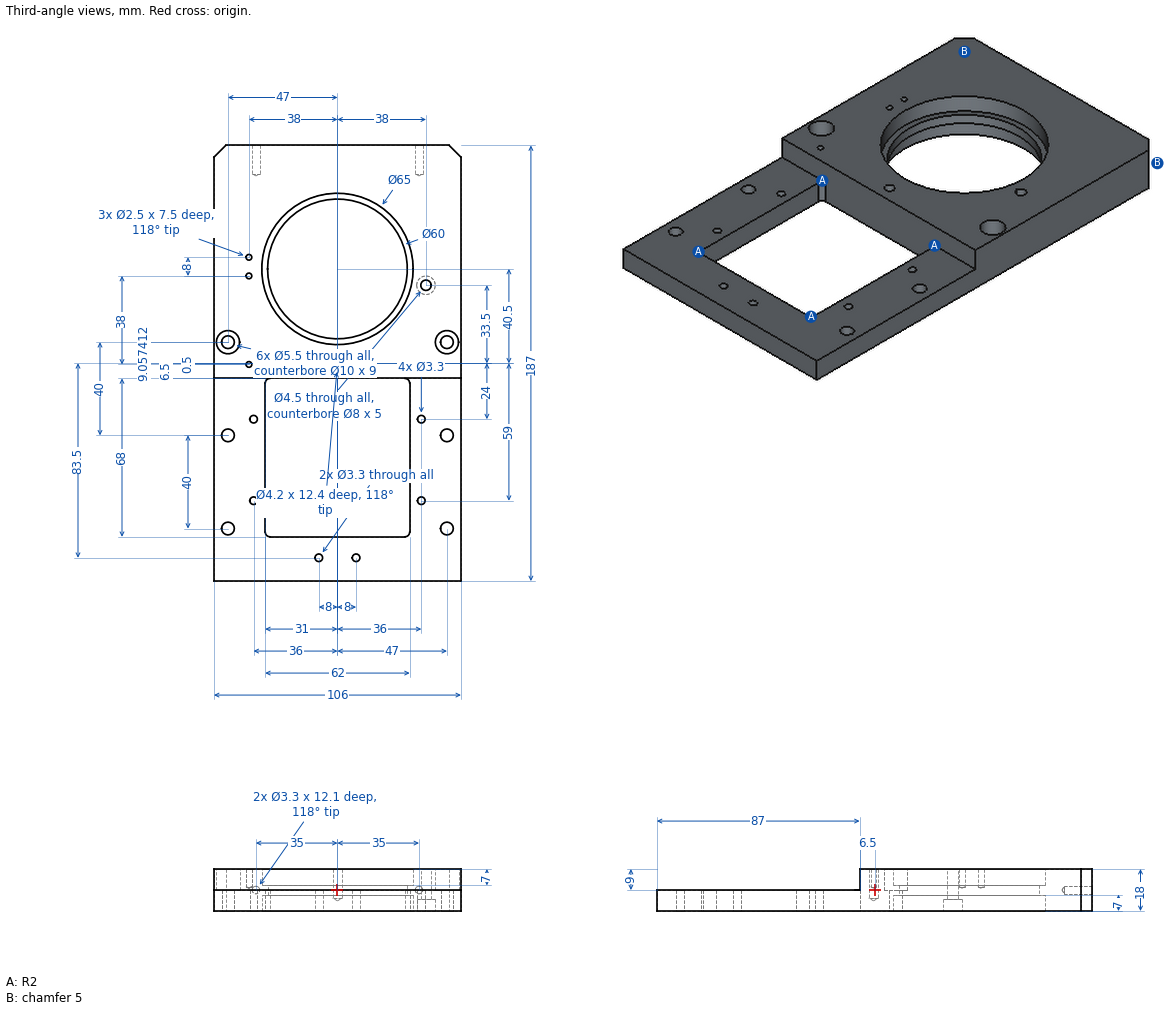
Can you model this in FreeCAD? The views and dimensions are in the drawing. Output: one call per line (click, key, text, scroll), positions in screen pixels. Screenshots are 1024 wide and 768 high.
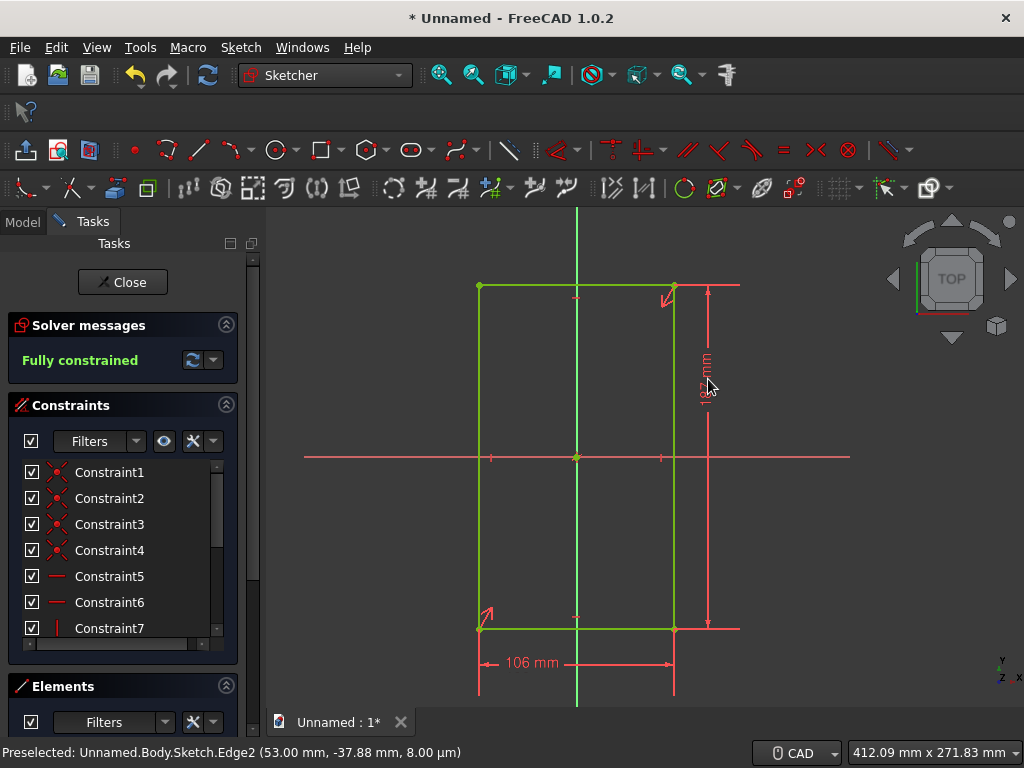
click(123, 282)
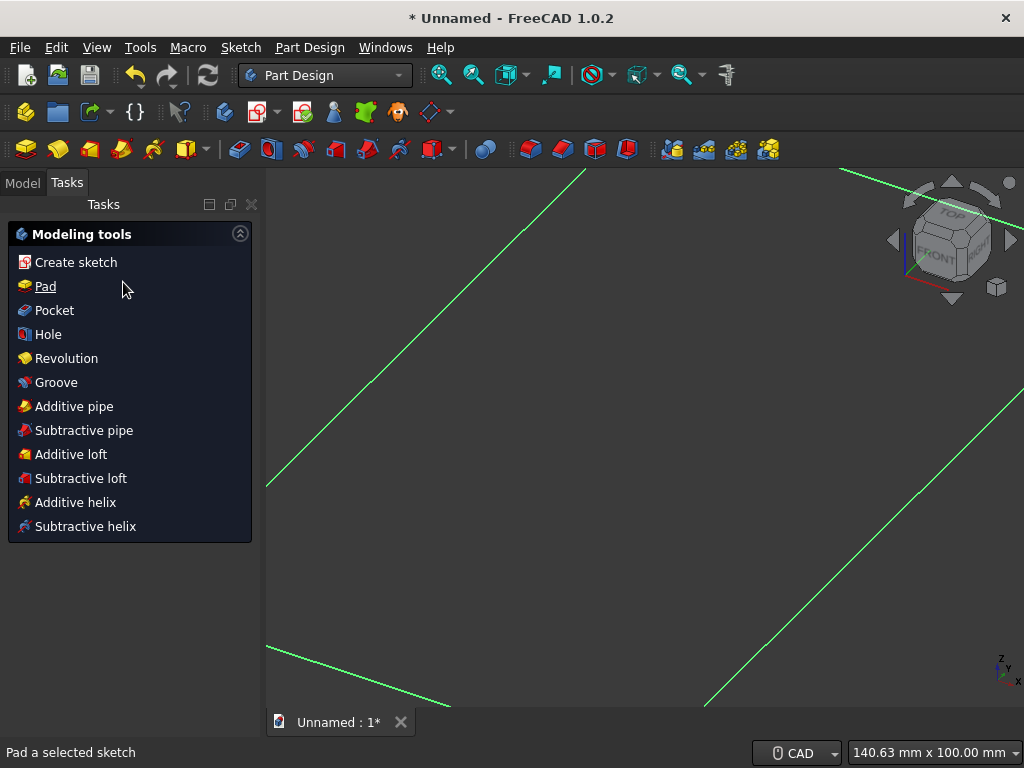
click(26, 150)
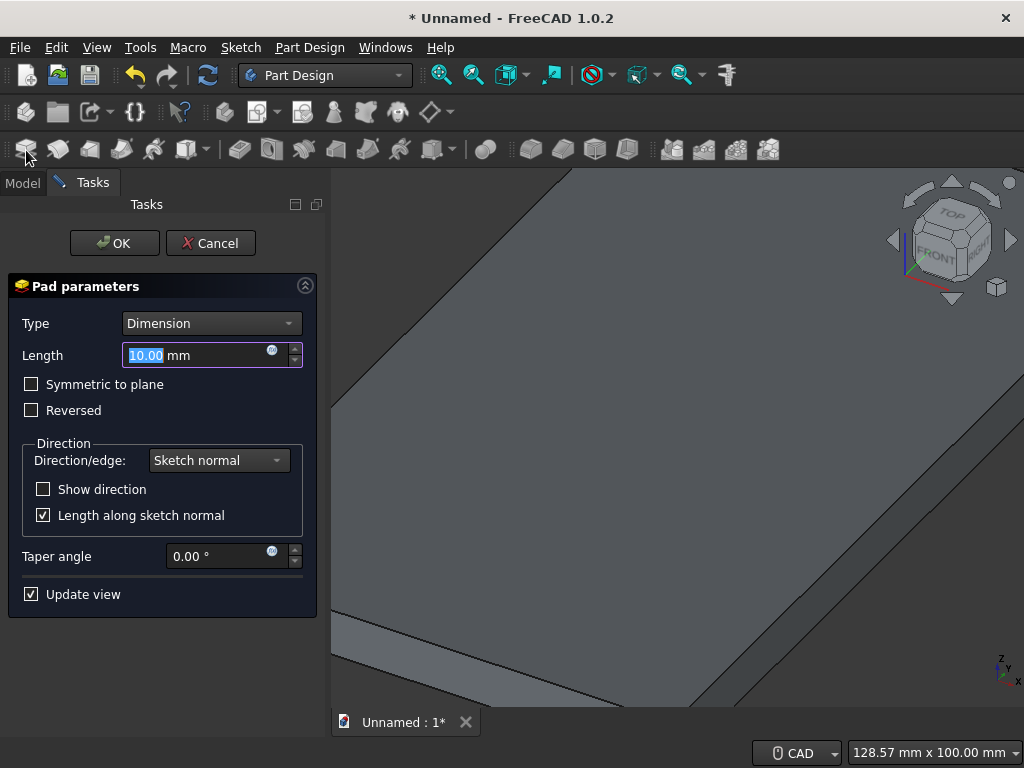
text(18)
key(Tab)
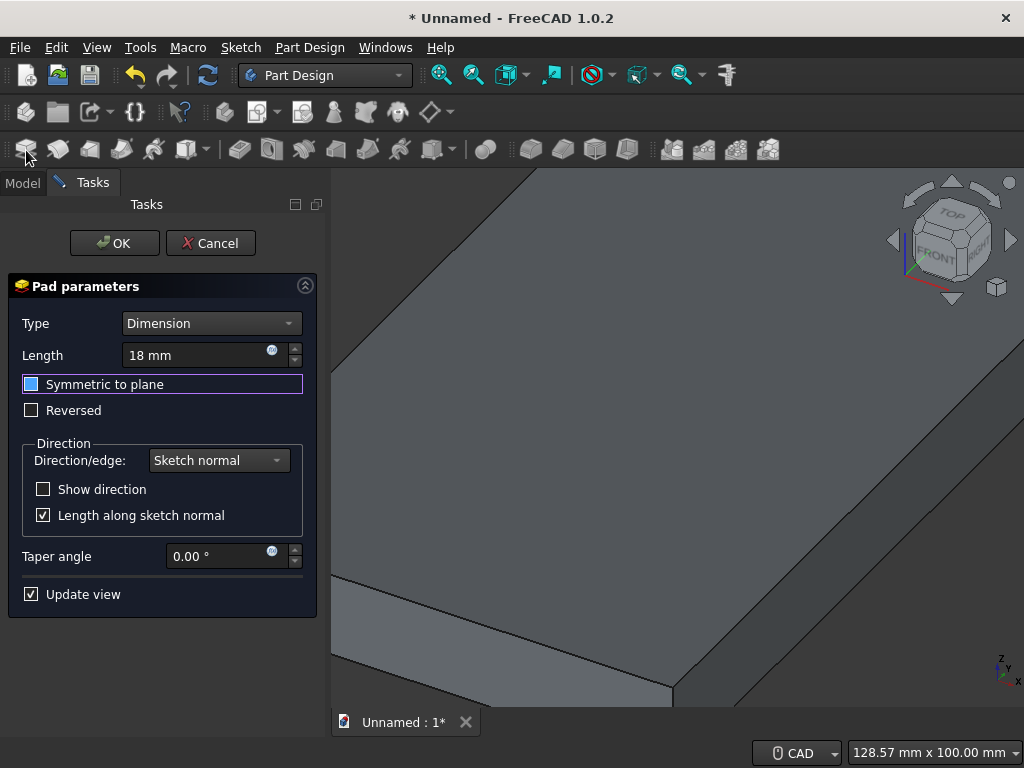
click(30, 384)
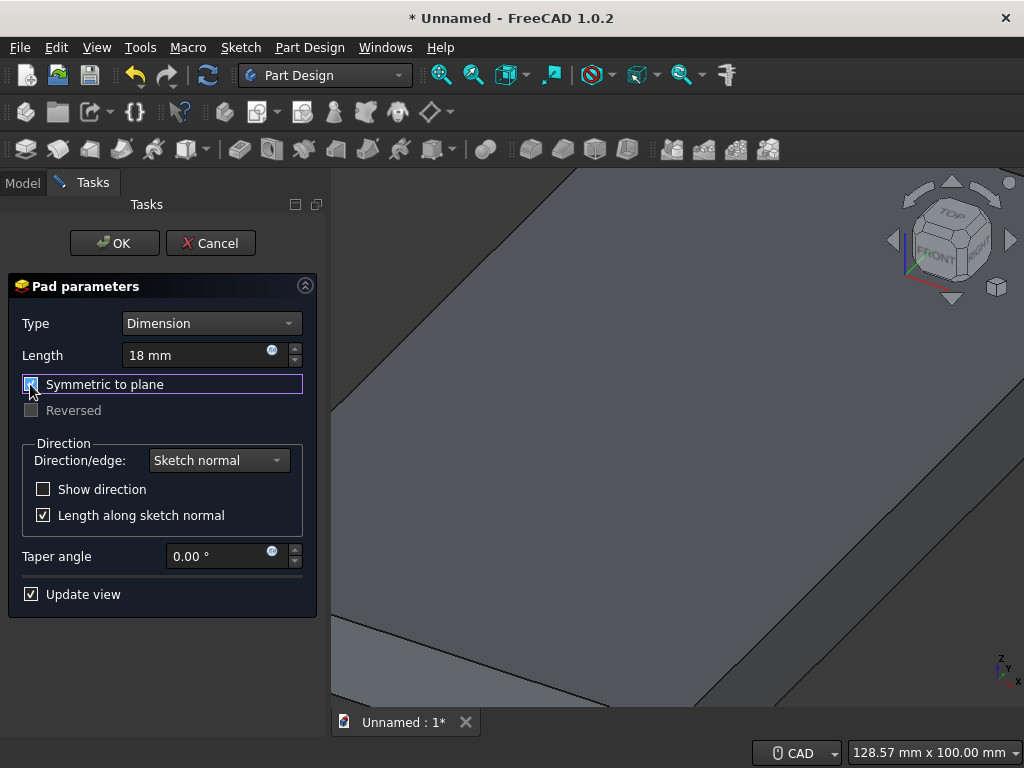
click(115, 243)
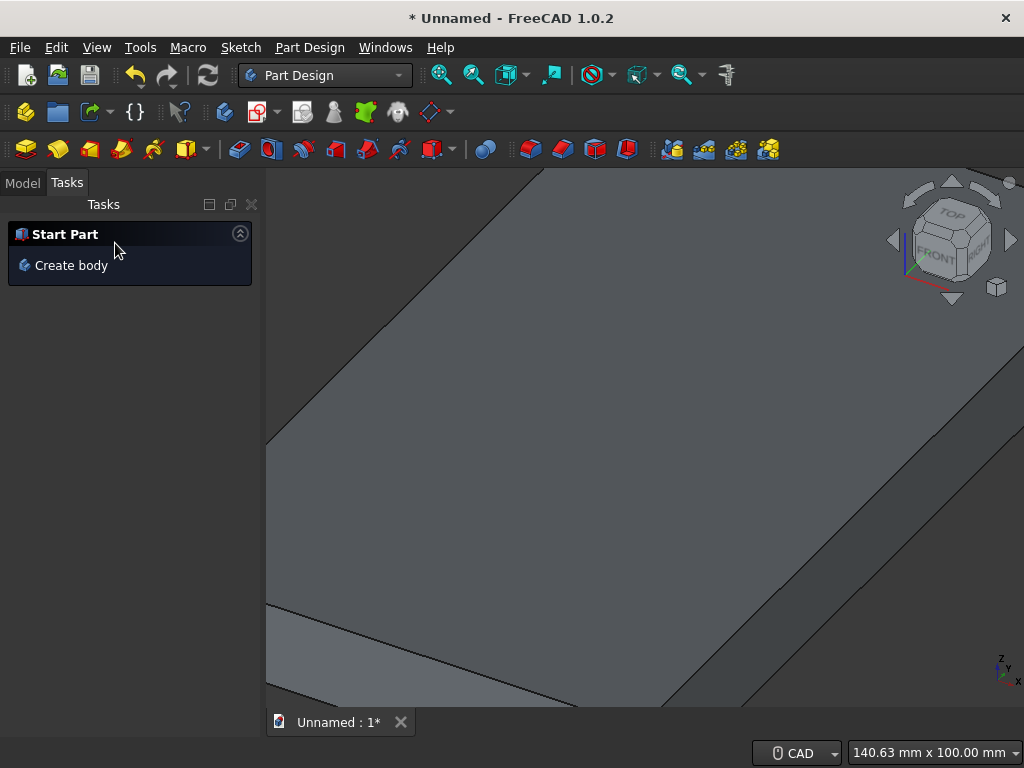
click(442, 76)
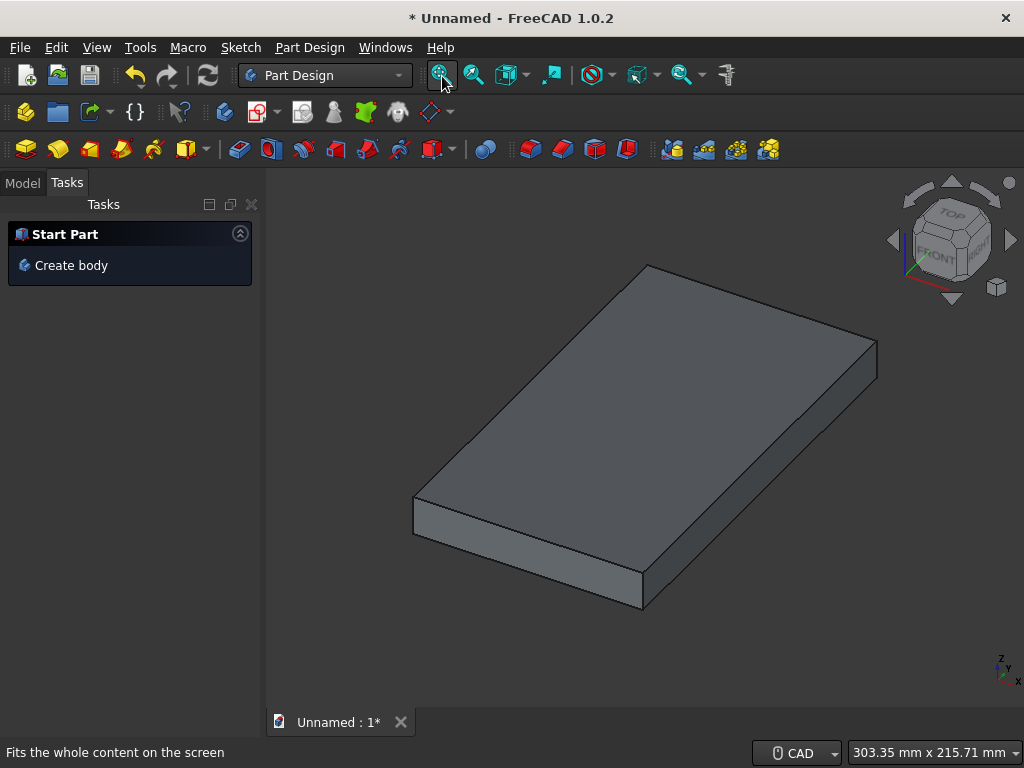
key(5)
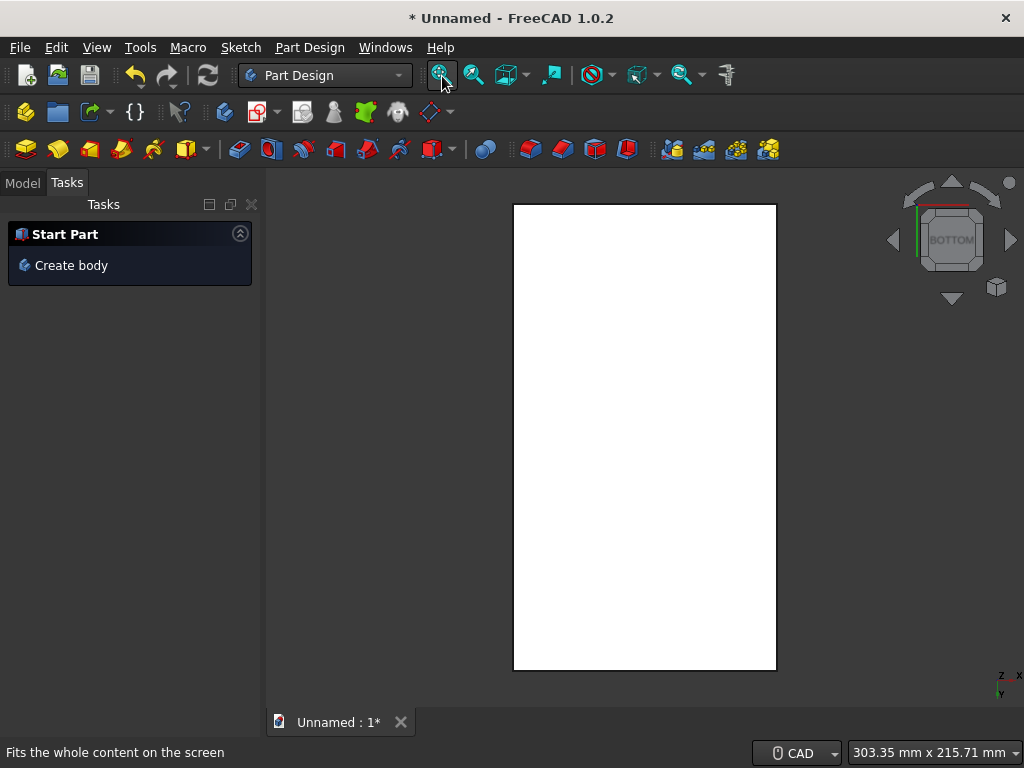
click(645, 503)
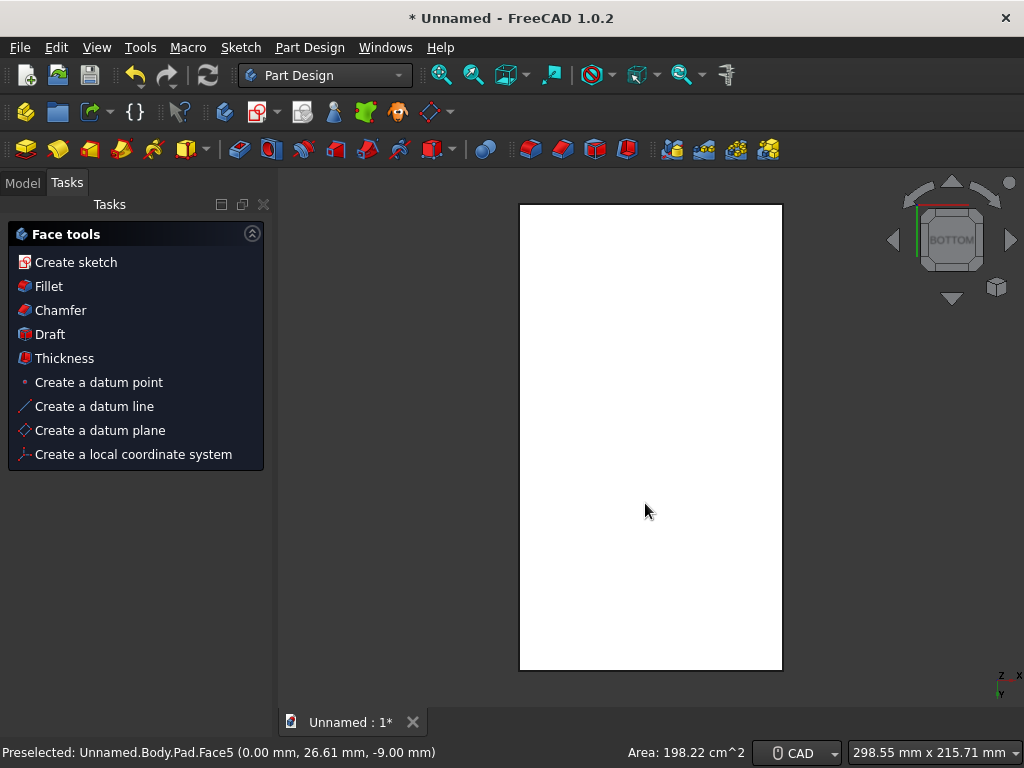
click(258, 112)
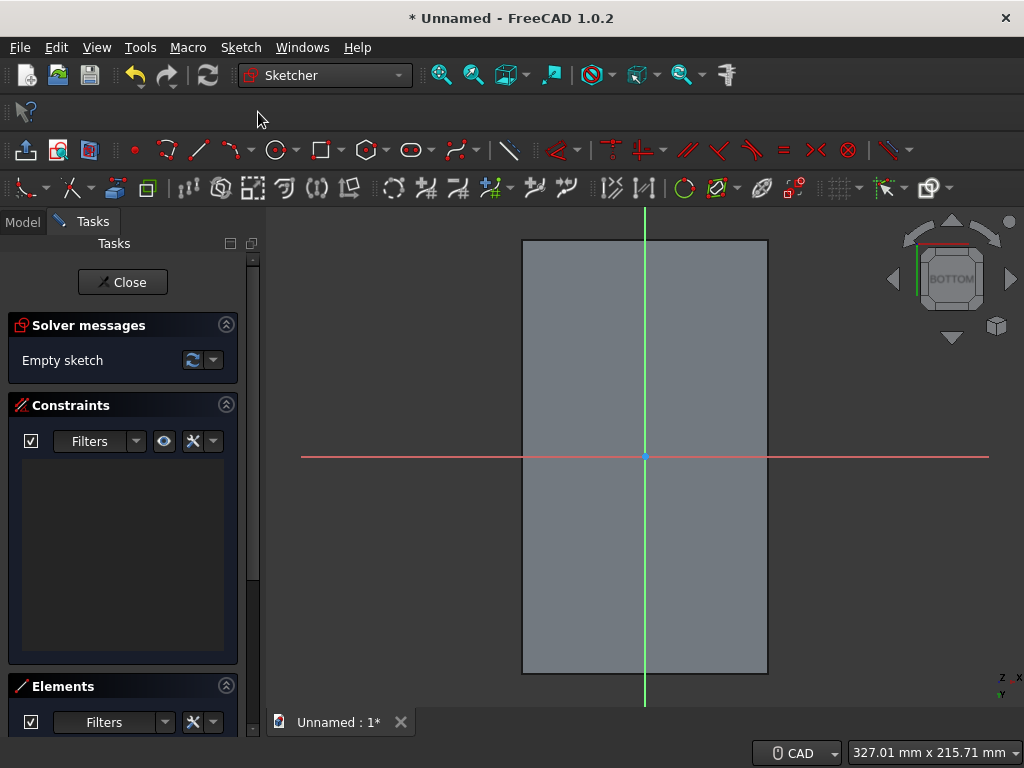
scroll(728, 638, up, 3)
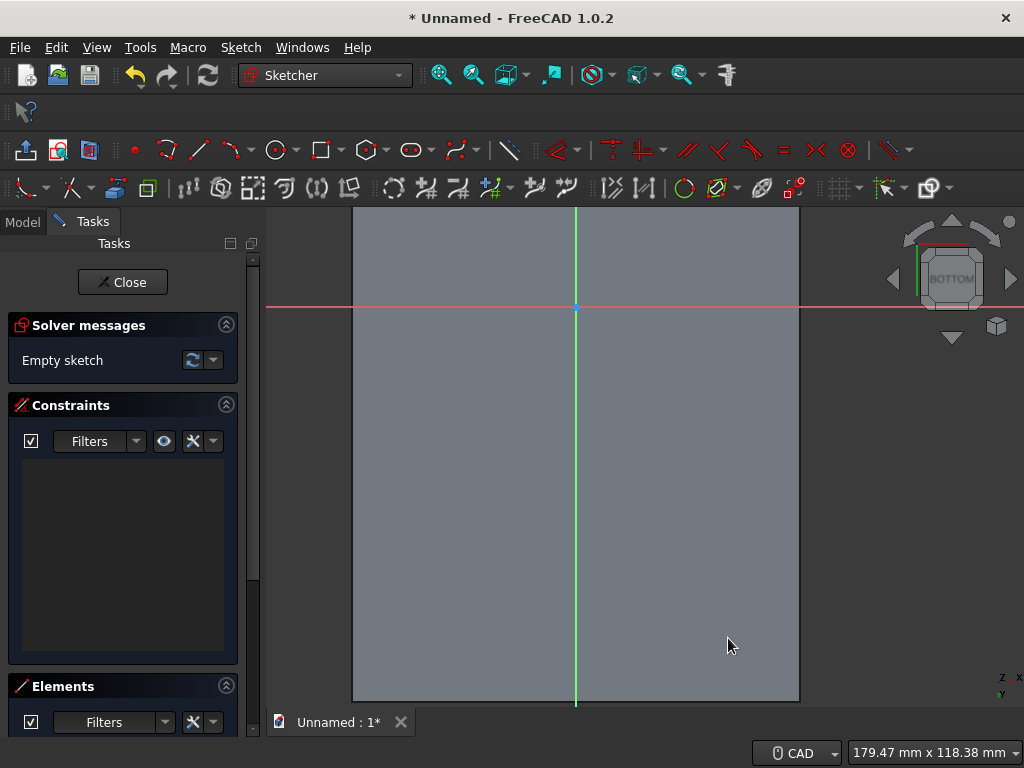
click(276, 150)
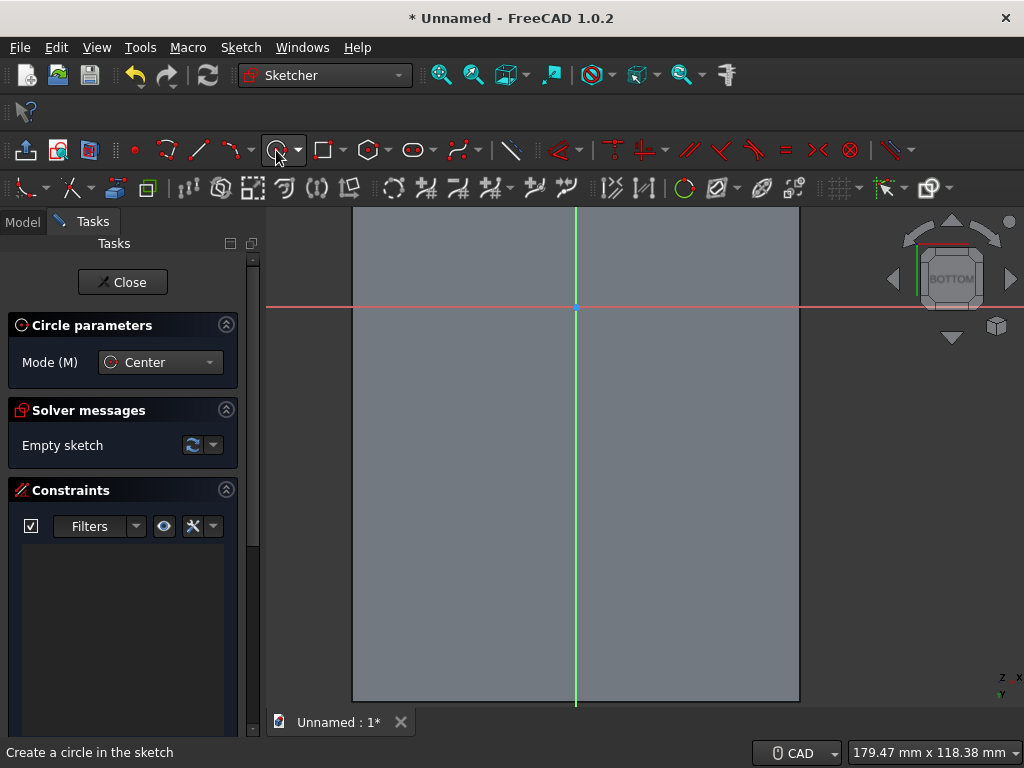
click(576, 479)
click(666, 389)
key(Escape)